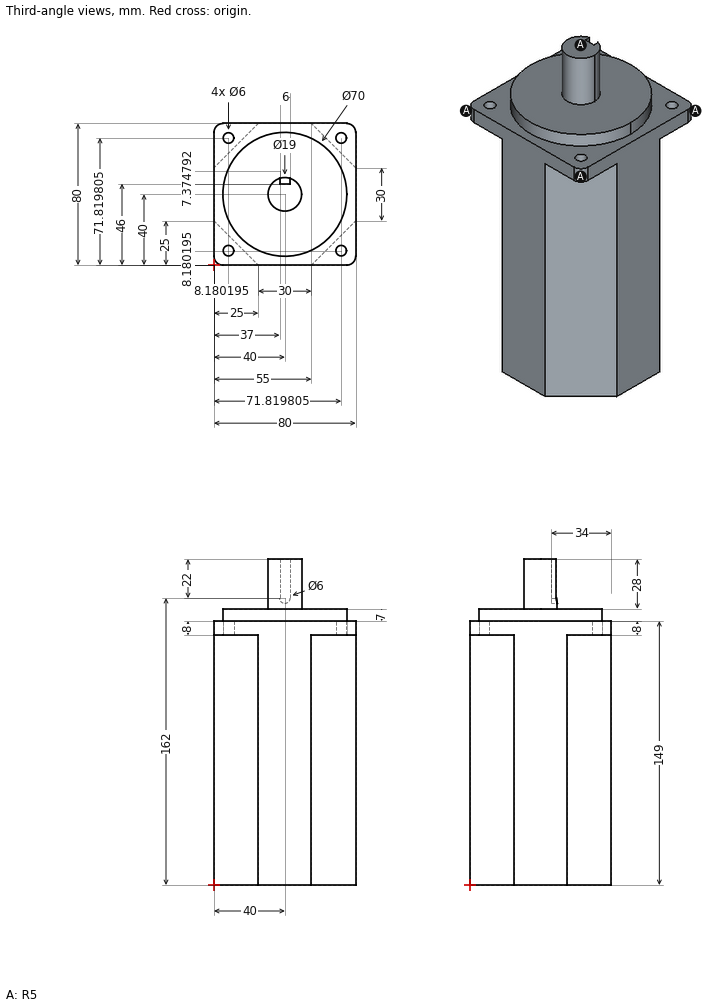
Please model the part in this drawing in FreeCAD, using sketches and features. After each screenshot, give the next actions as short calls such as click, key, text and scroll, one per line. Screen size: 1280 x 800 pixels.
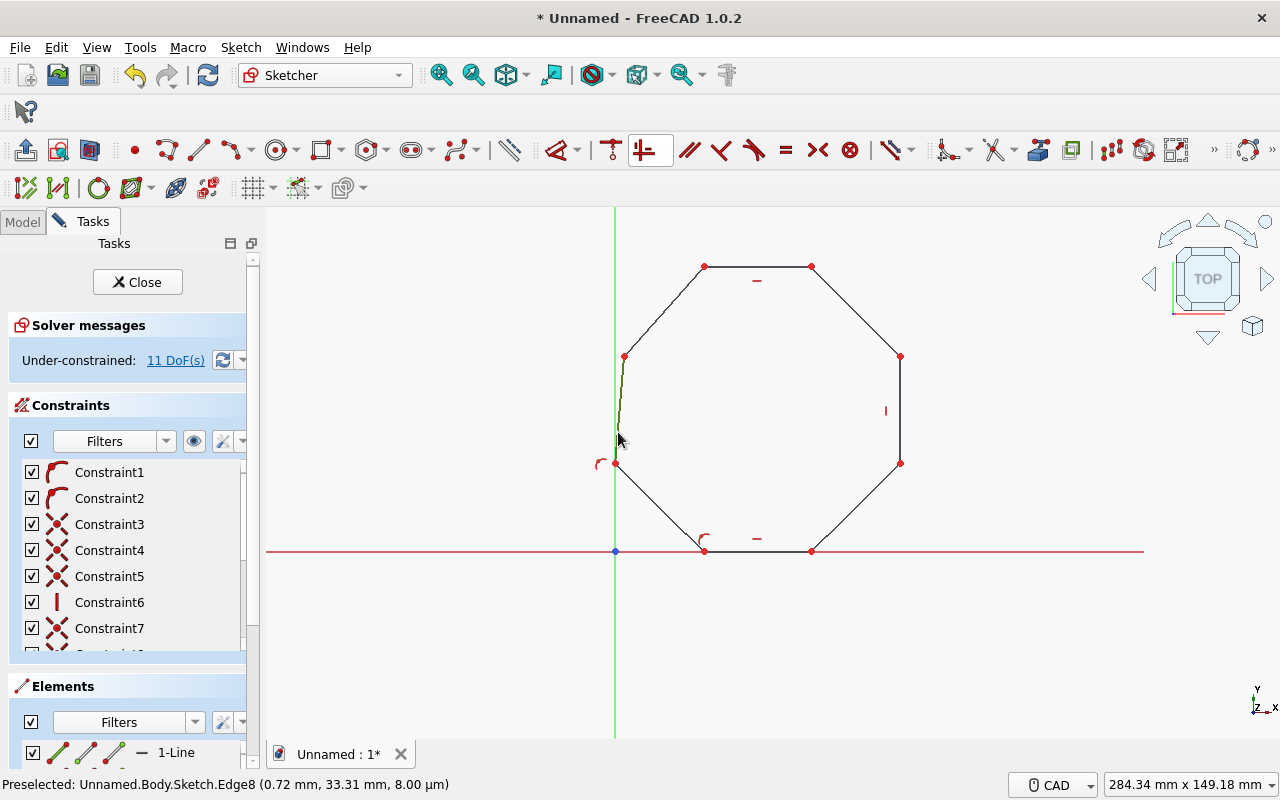
click(668, 150)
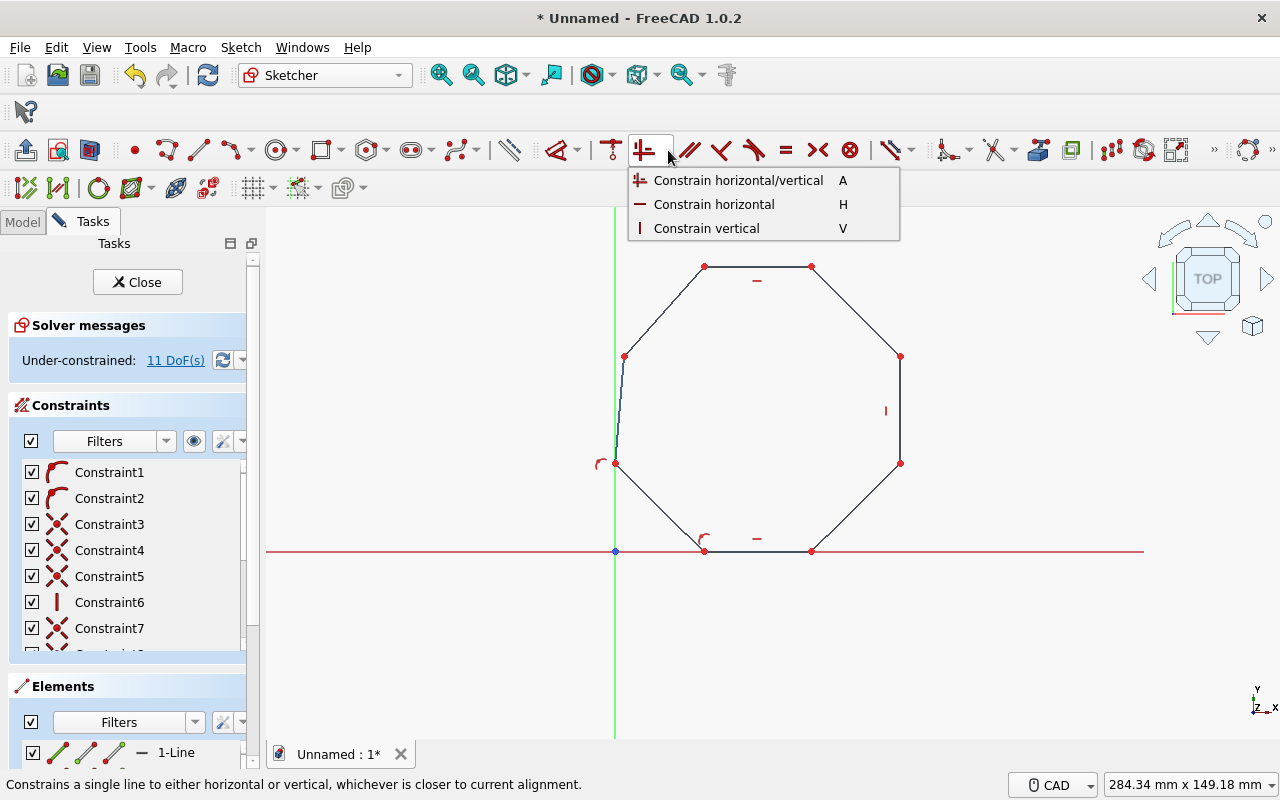
click(764, 228)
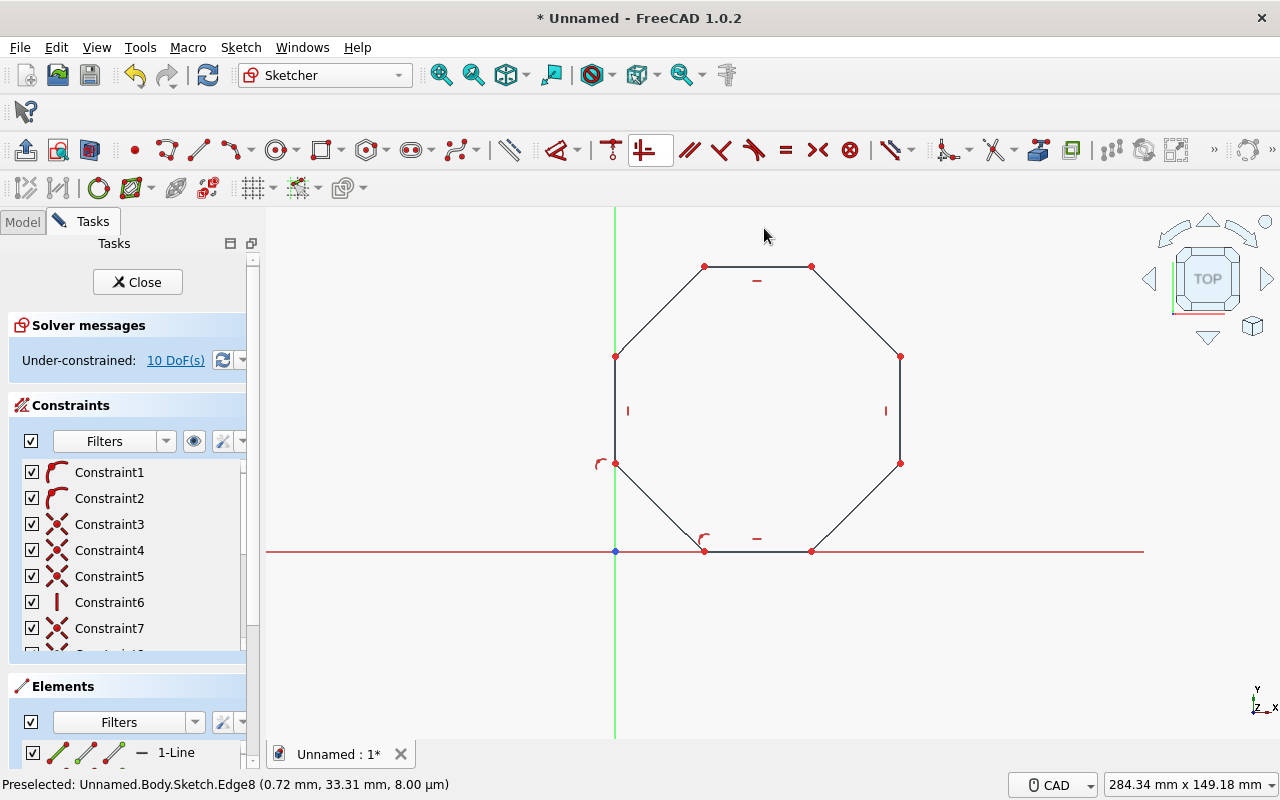
key(d)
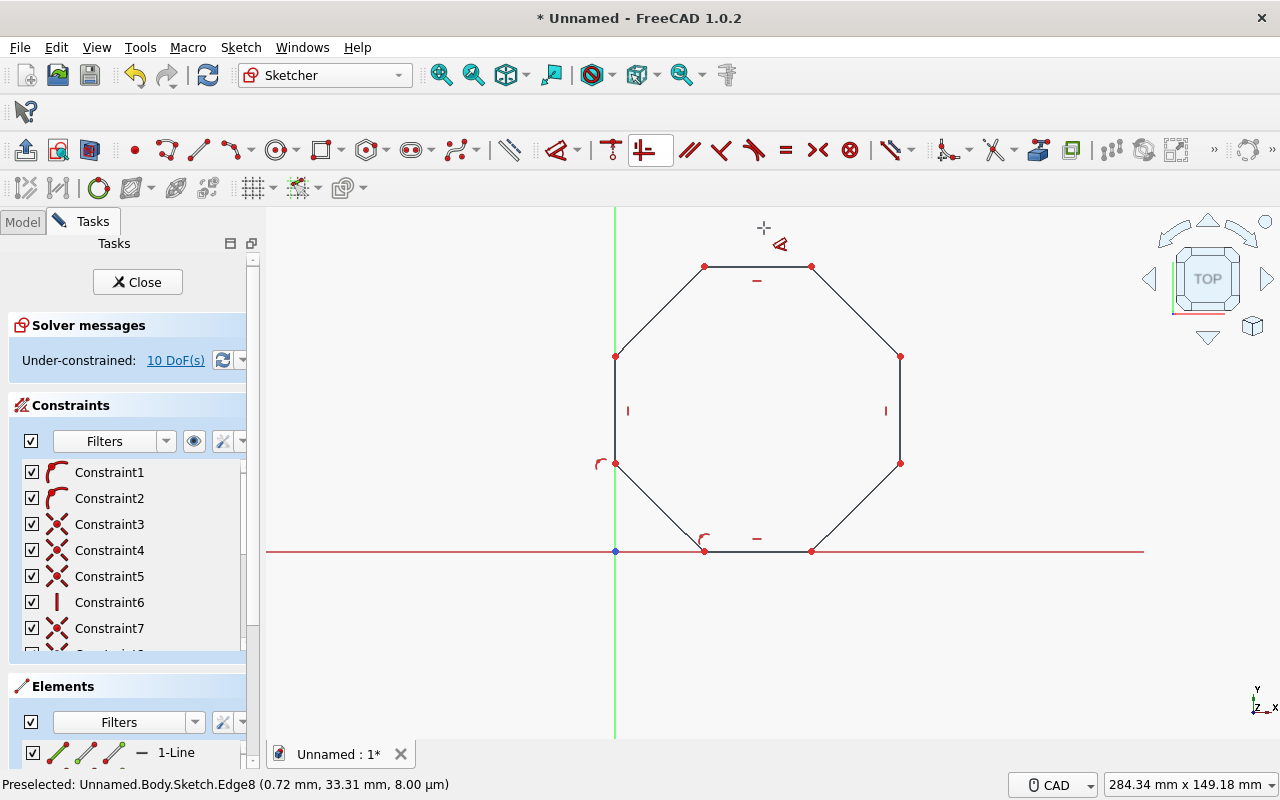
click(736, 552)
click(758, 586)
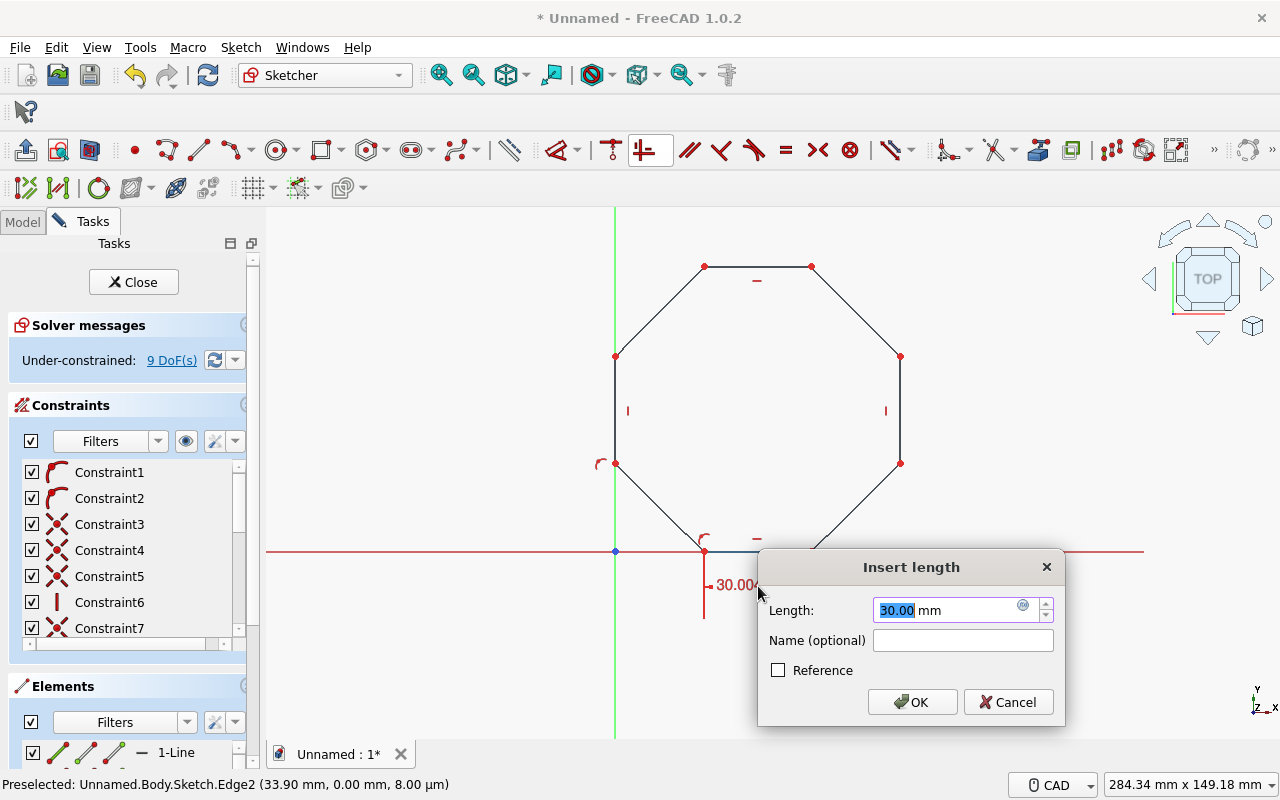
text(30)
key(Return)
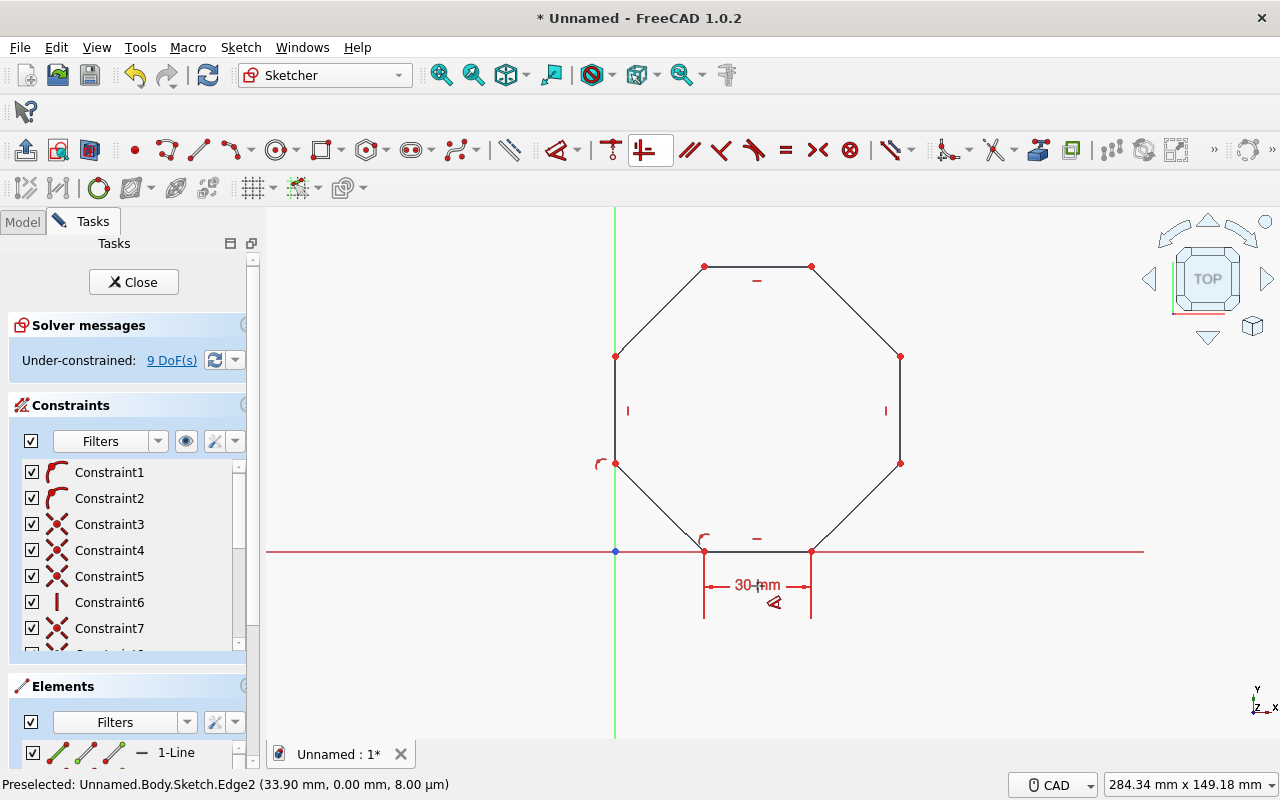
click(900, 432)
click(934, 411)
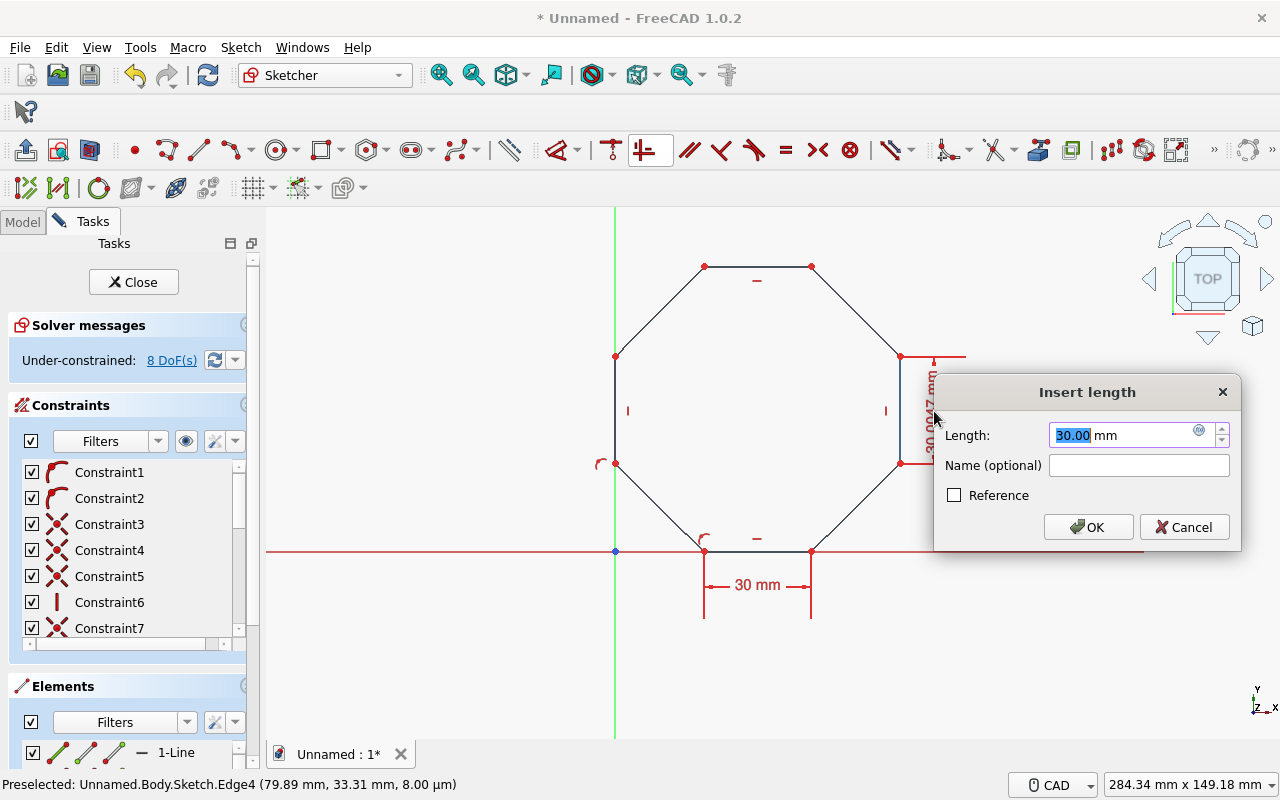
text(30)
key(Return)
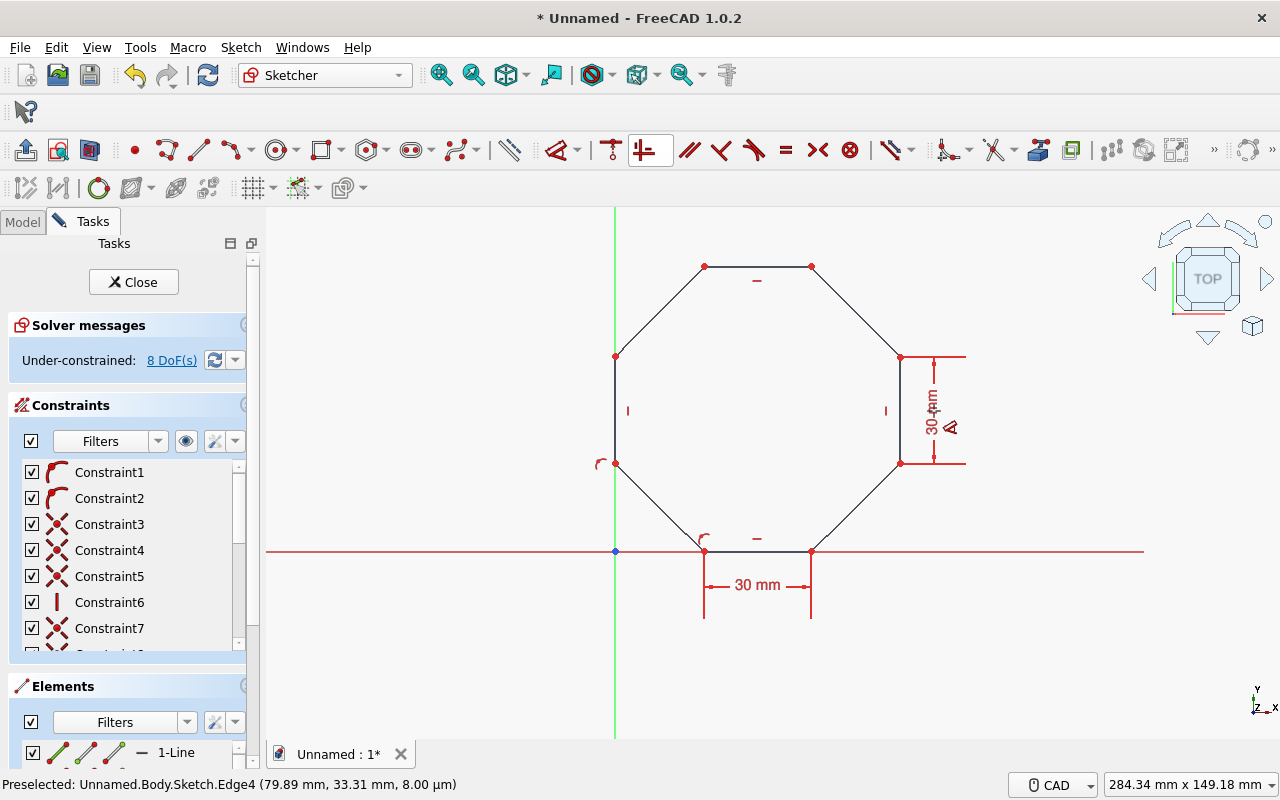
click(779, 267)
click(758, 301)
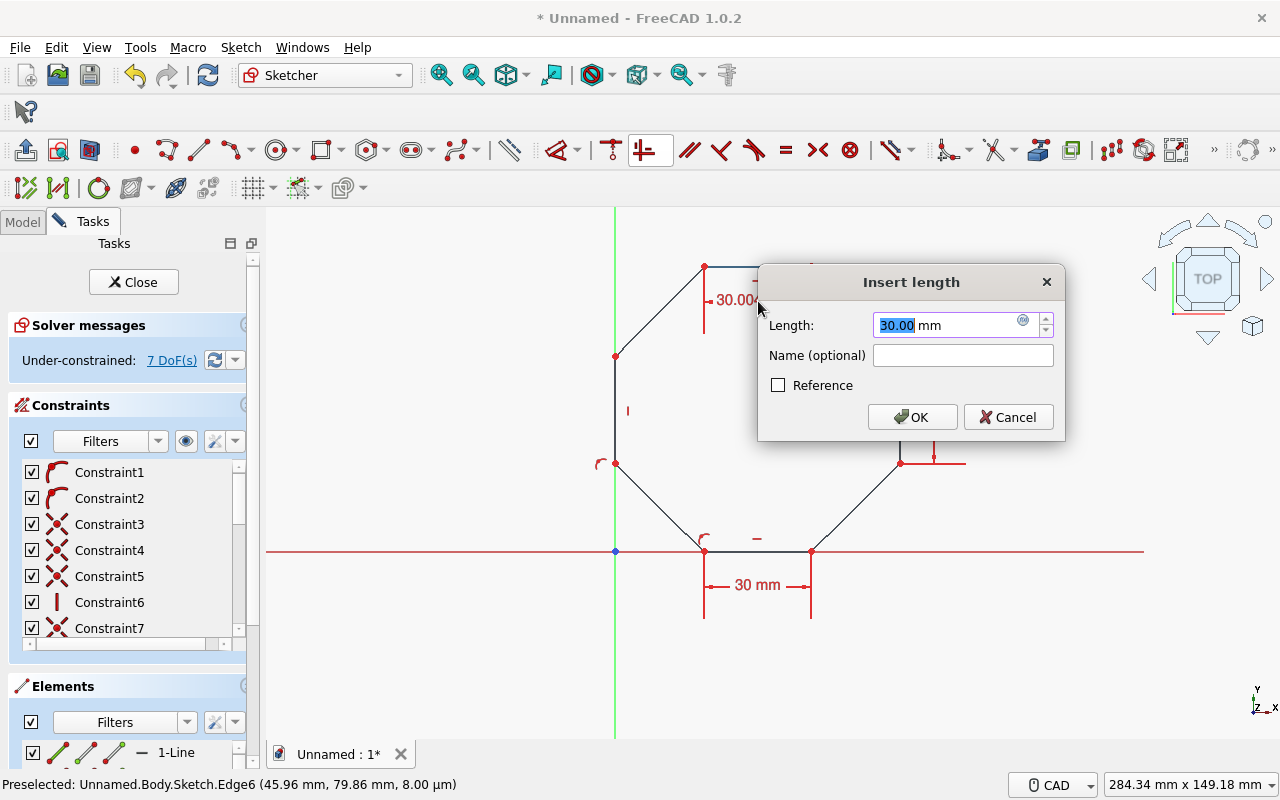
text(30)
key(Return)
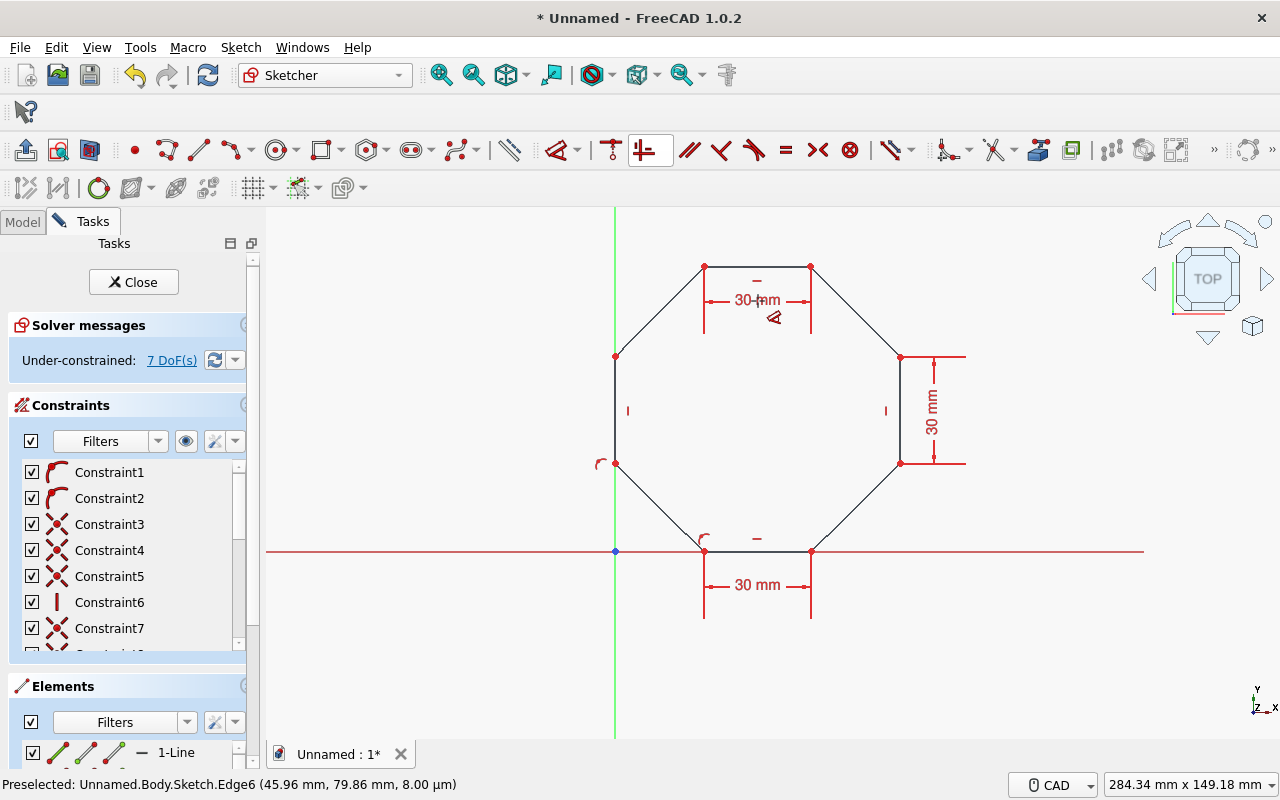
click(615, 389)
click(581, 411)